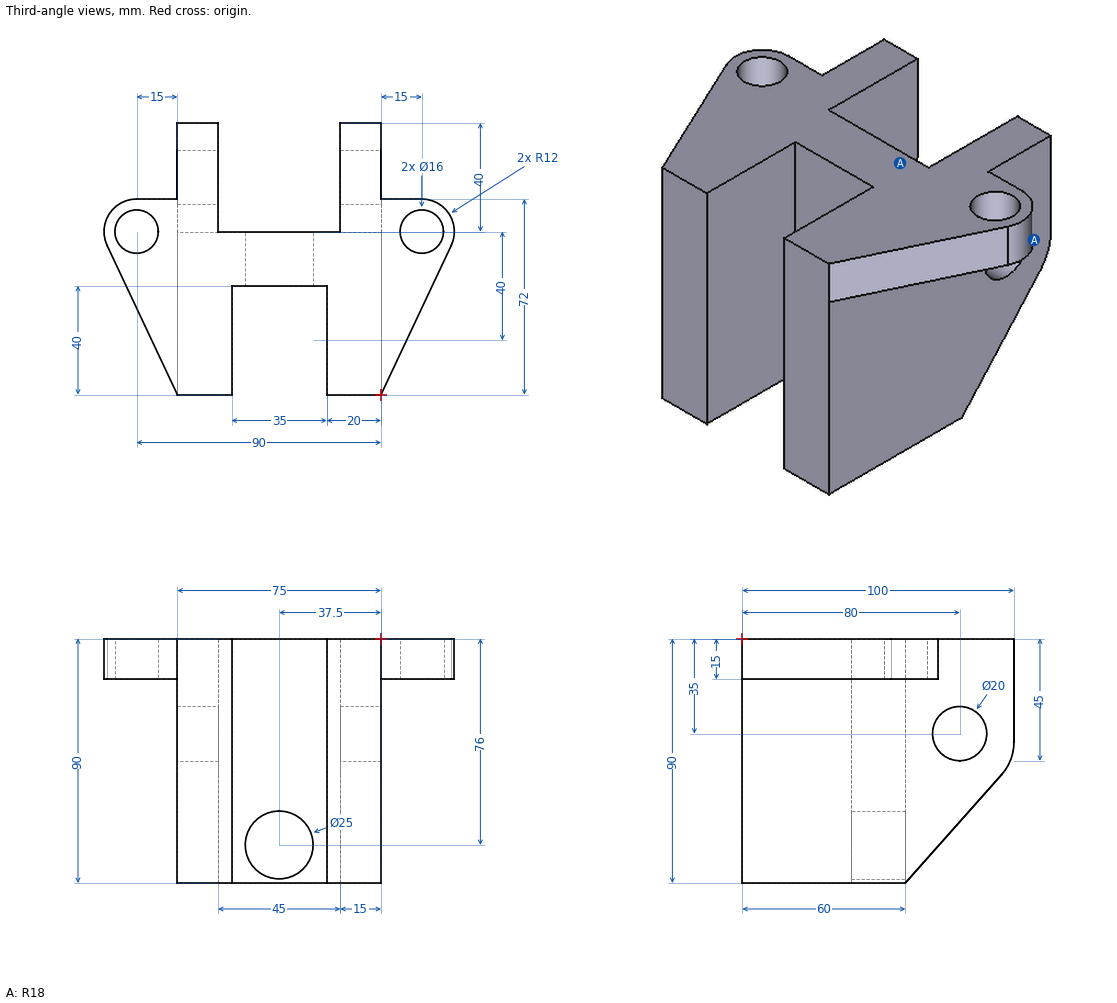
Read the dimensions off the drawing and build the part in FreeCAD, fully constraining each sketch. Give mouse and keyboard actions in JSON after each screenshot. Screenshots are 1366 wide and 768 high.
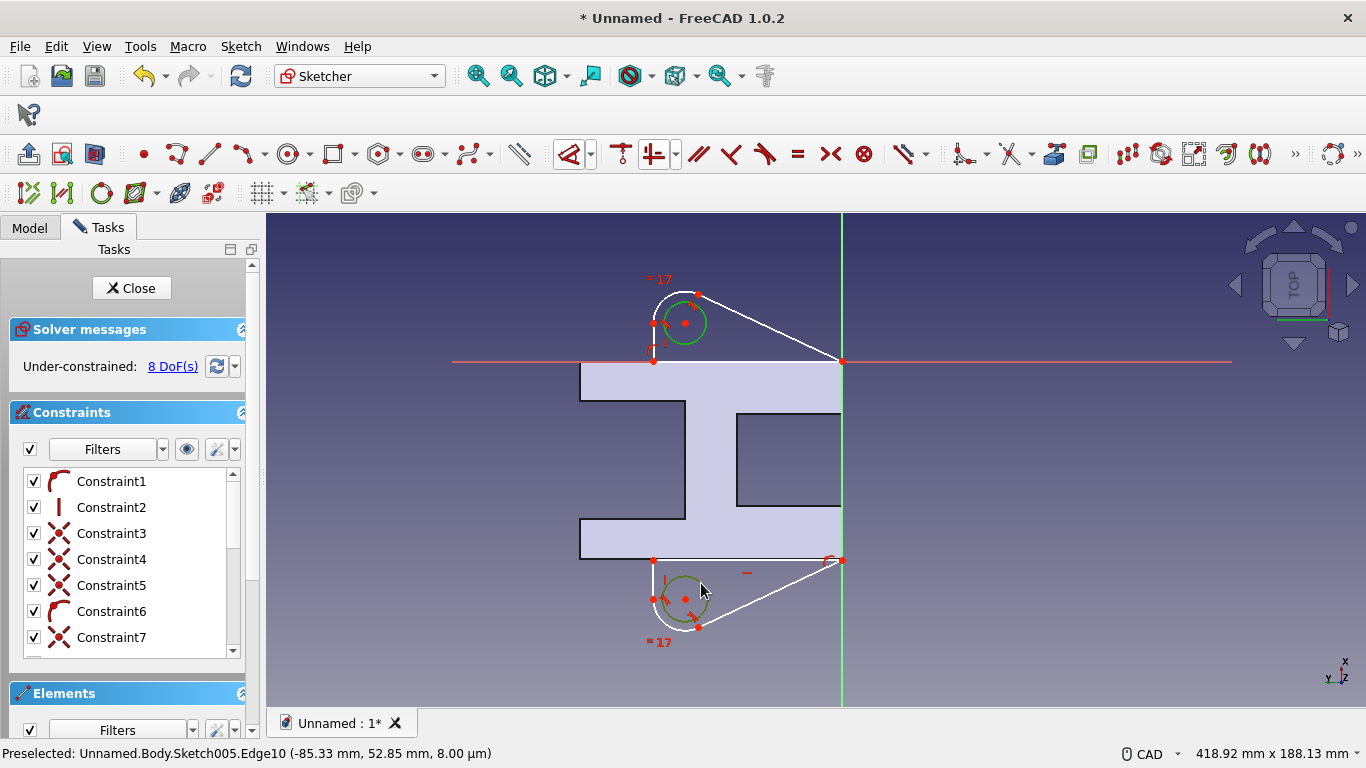
{"action": "key", "text": "e"}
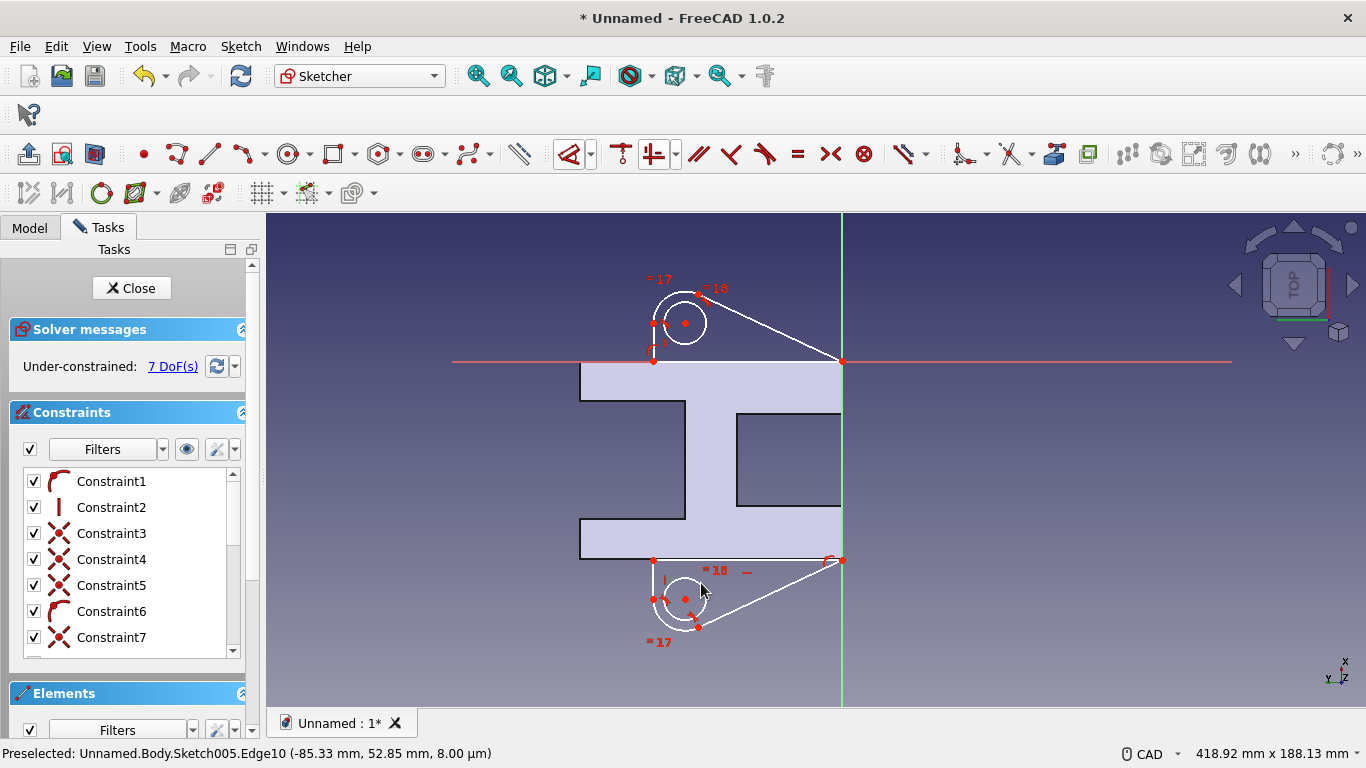
{"action": "scroll", "coordinate": [680, 292], "scroll_direction": "up", "scroll_amount": 2}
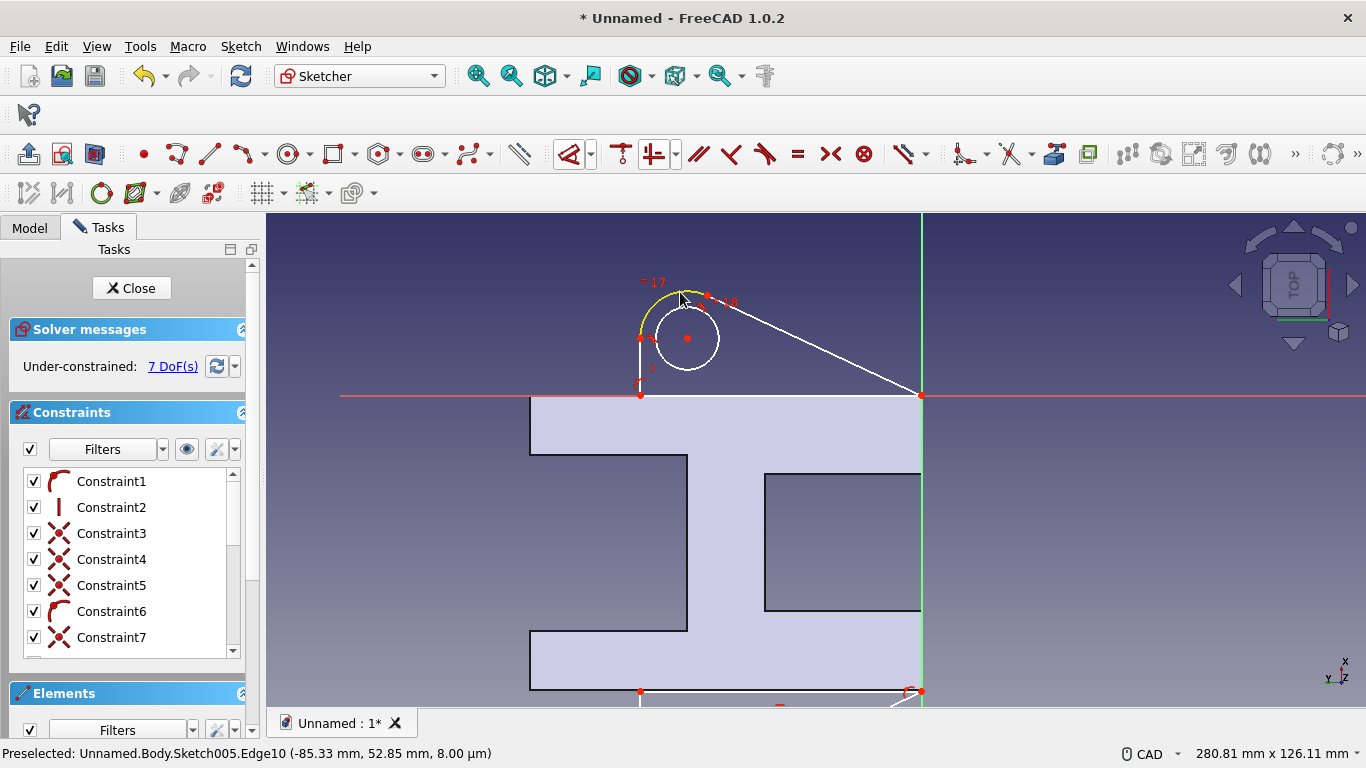
{"action": "left_click", "coordinate": [680, 292]}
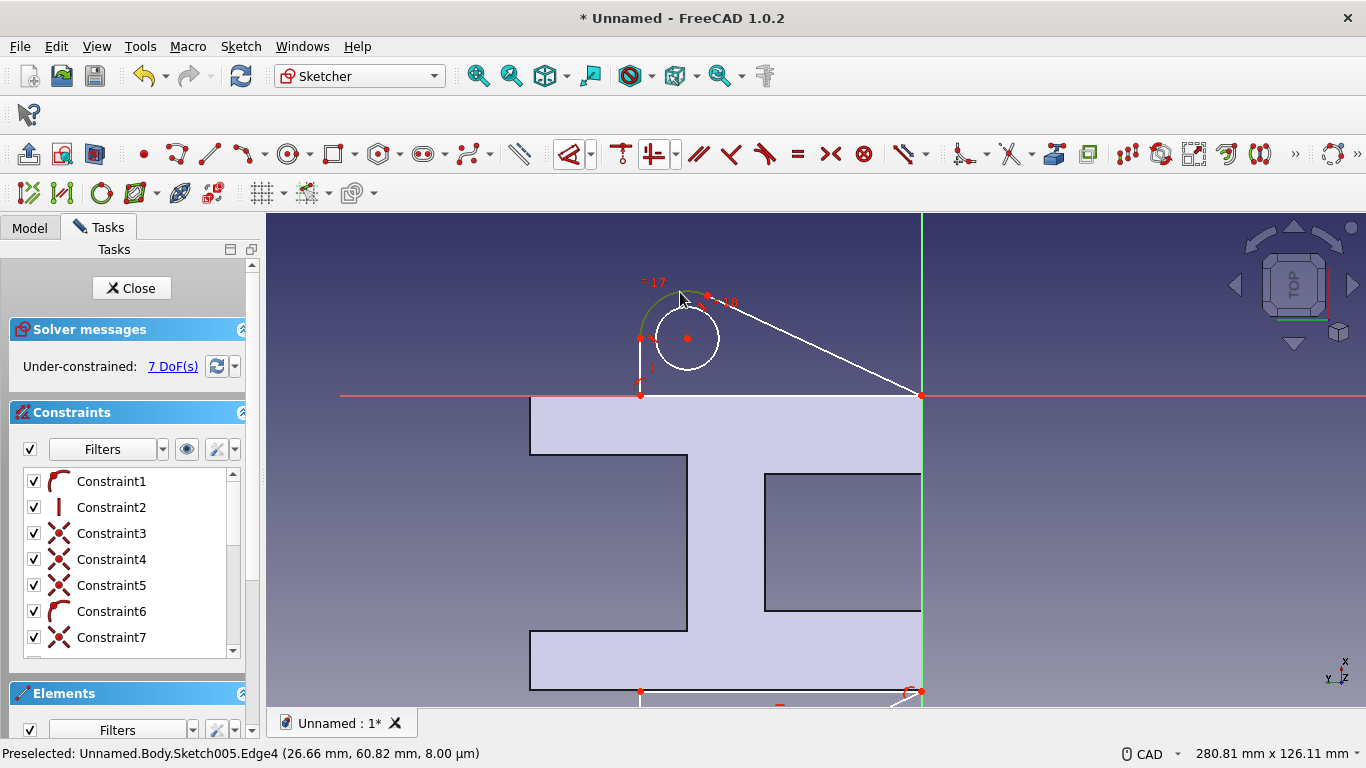
{"action": "key", "text": "k r"}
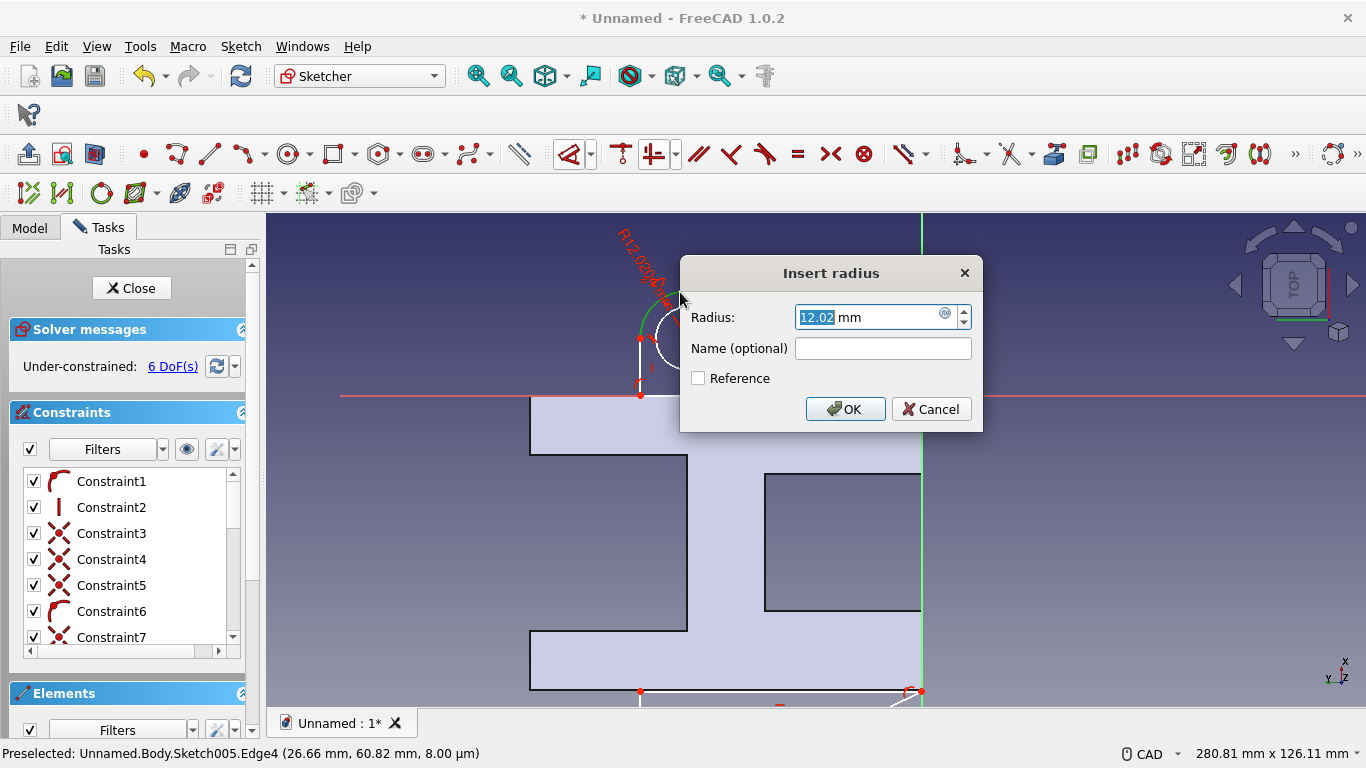
{"action": "type", "text": "12"}
{"action": "key", "text": "Return"}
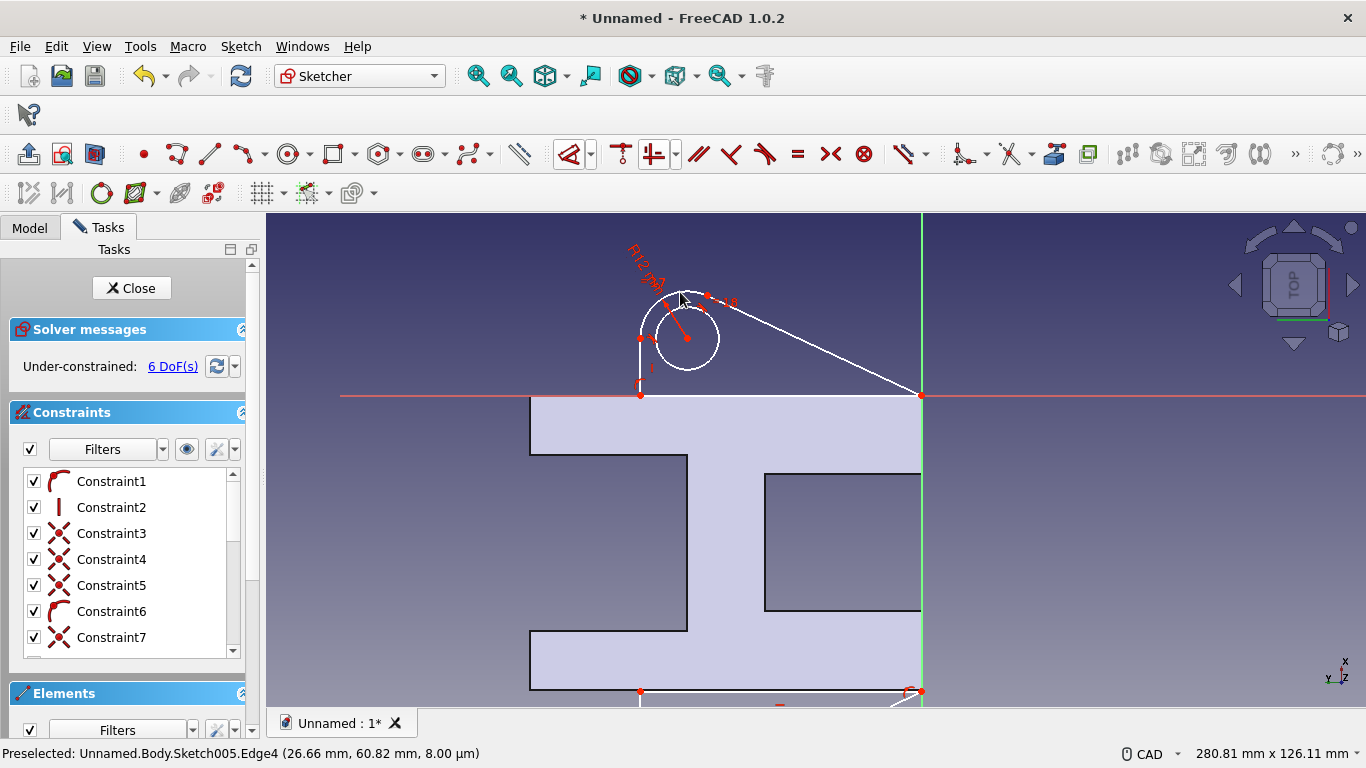
{"action": "left_click", "coordinate": [710, 316]}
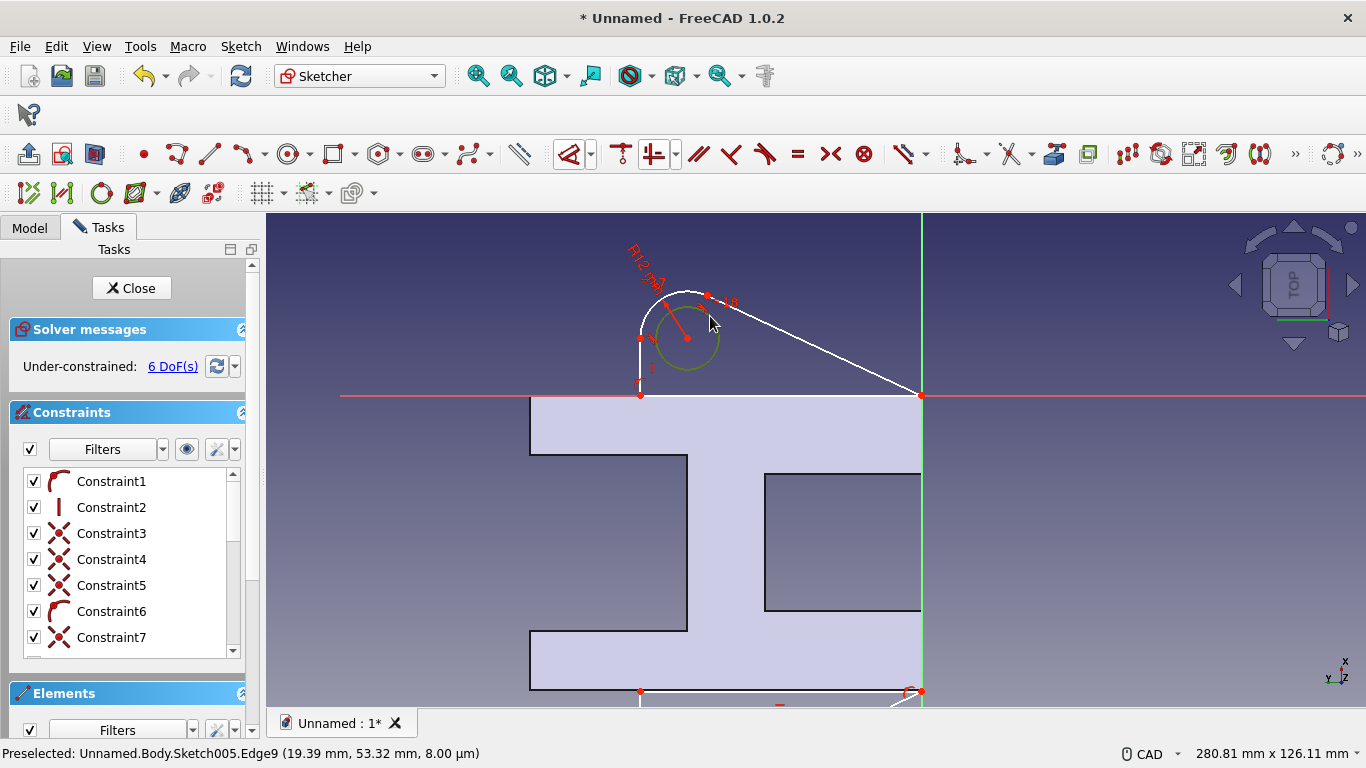
{"action": "key", "text": "k o"}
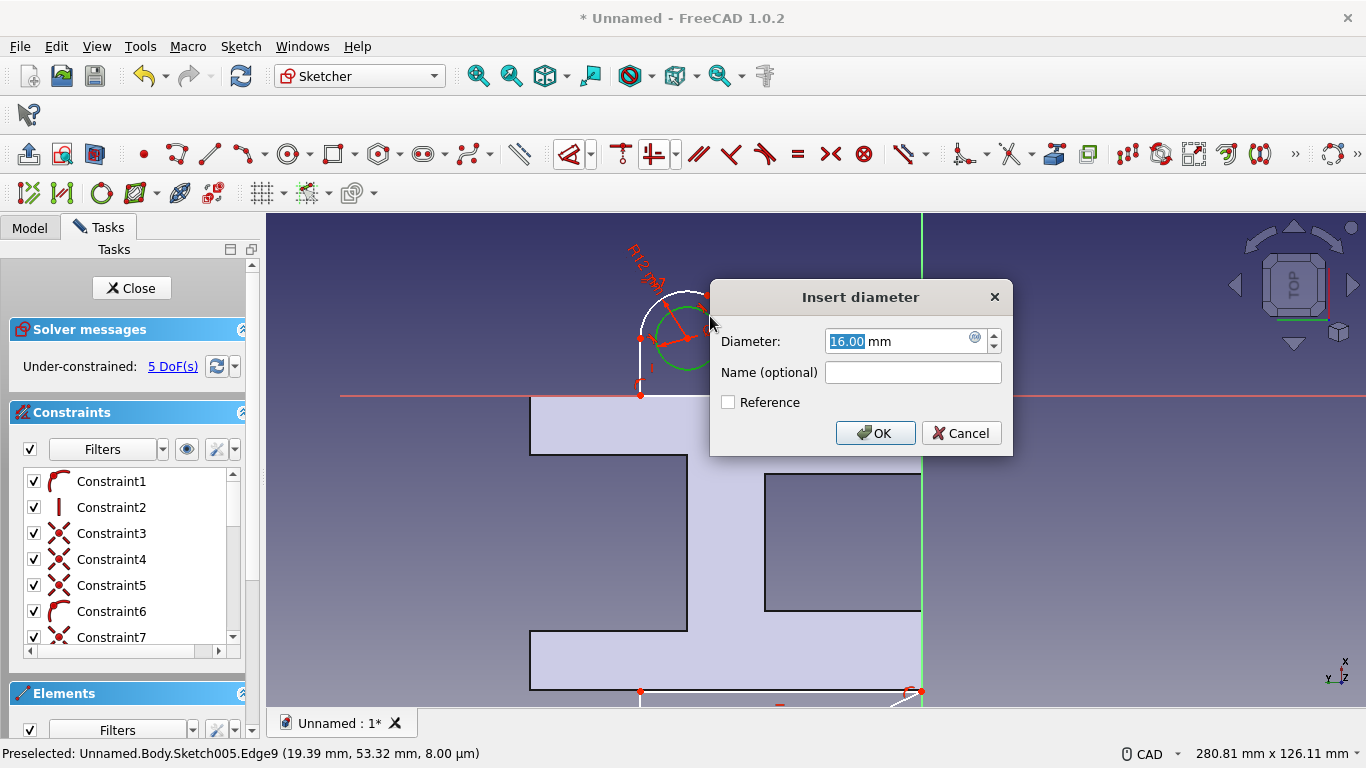
{"action": "type", "text": "16"}
{"action": "key", "text": "Return"}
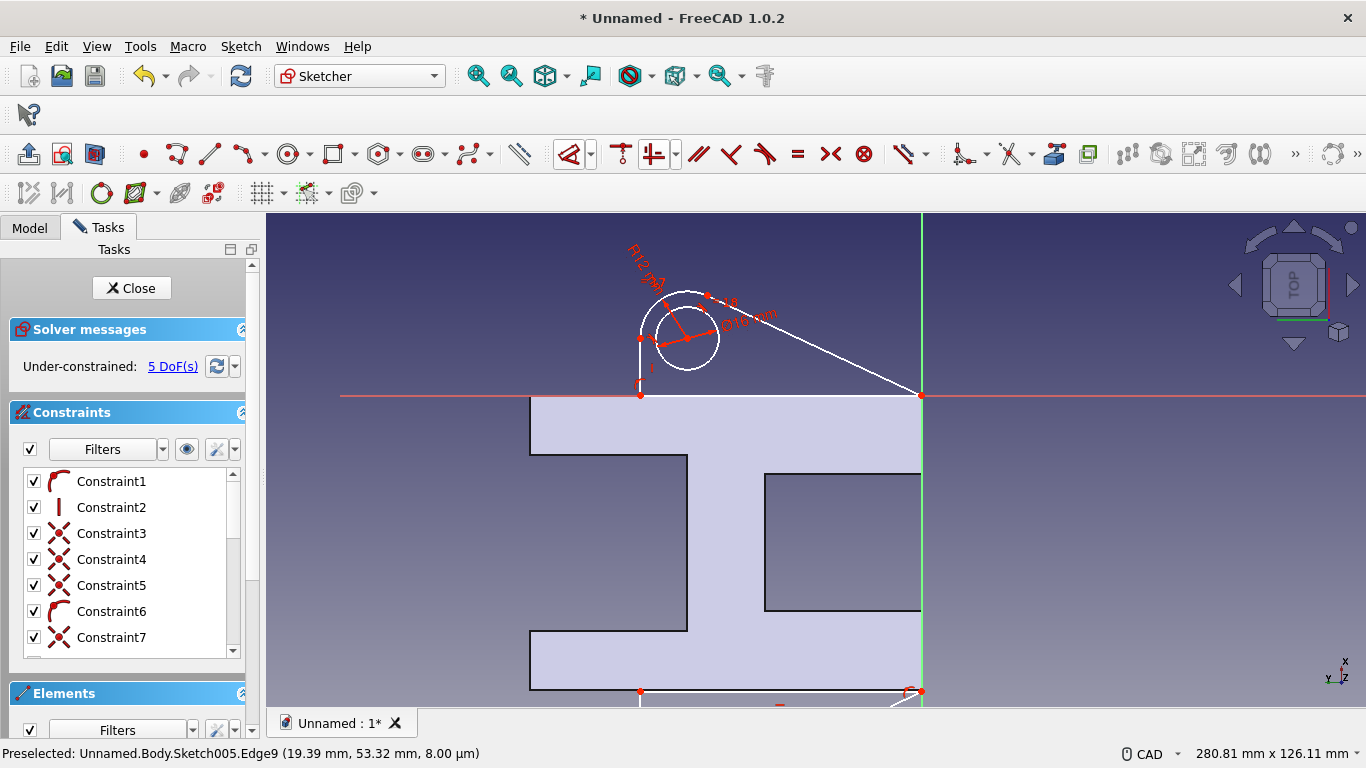
{"action": "left_click", "coordinate": [640, 356]}